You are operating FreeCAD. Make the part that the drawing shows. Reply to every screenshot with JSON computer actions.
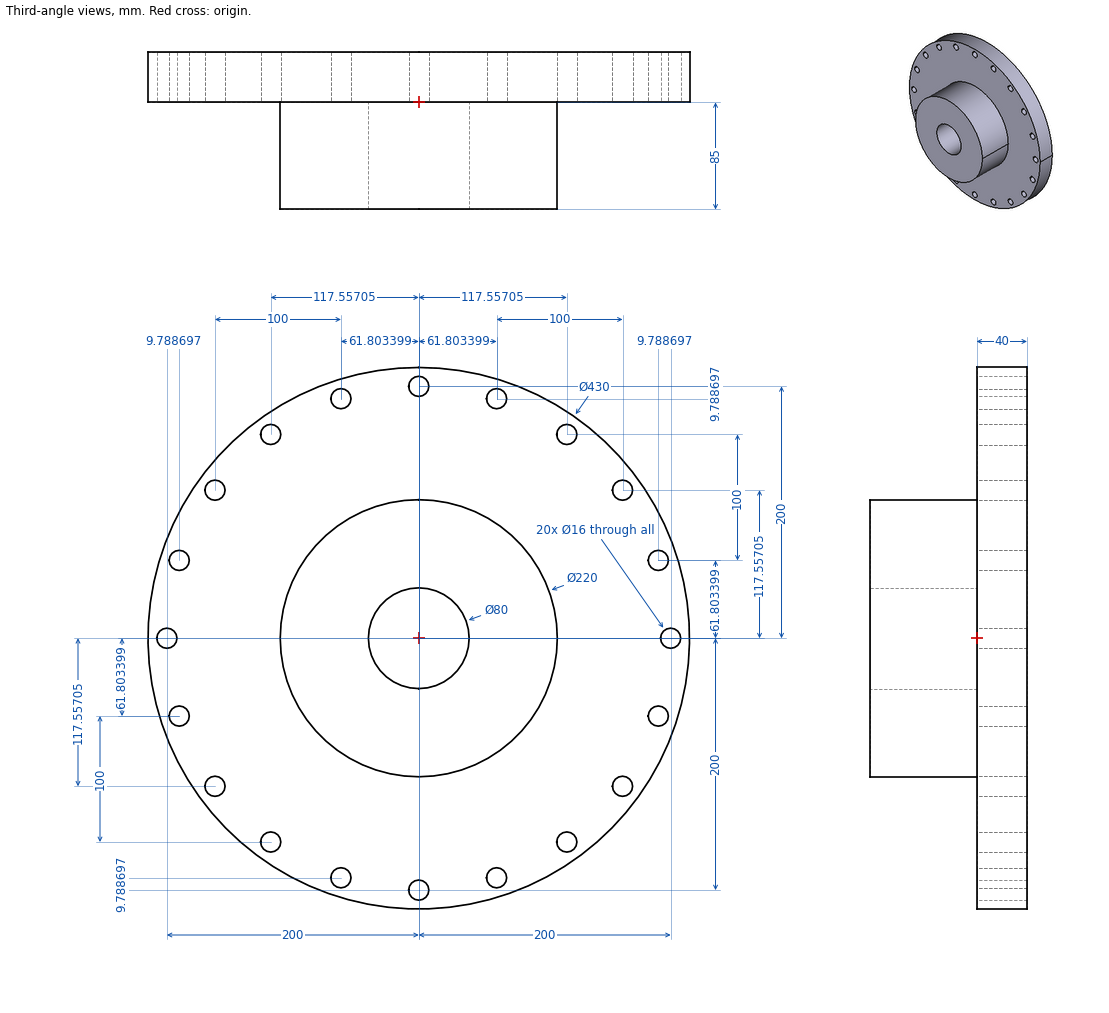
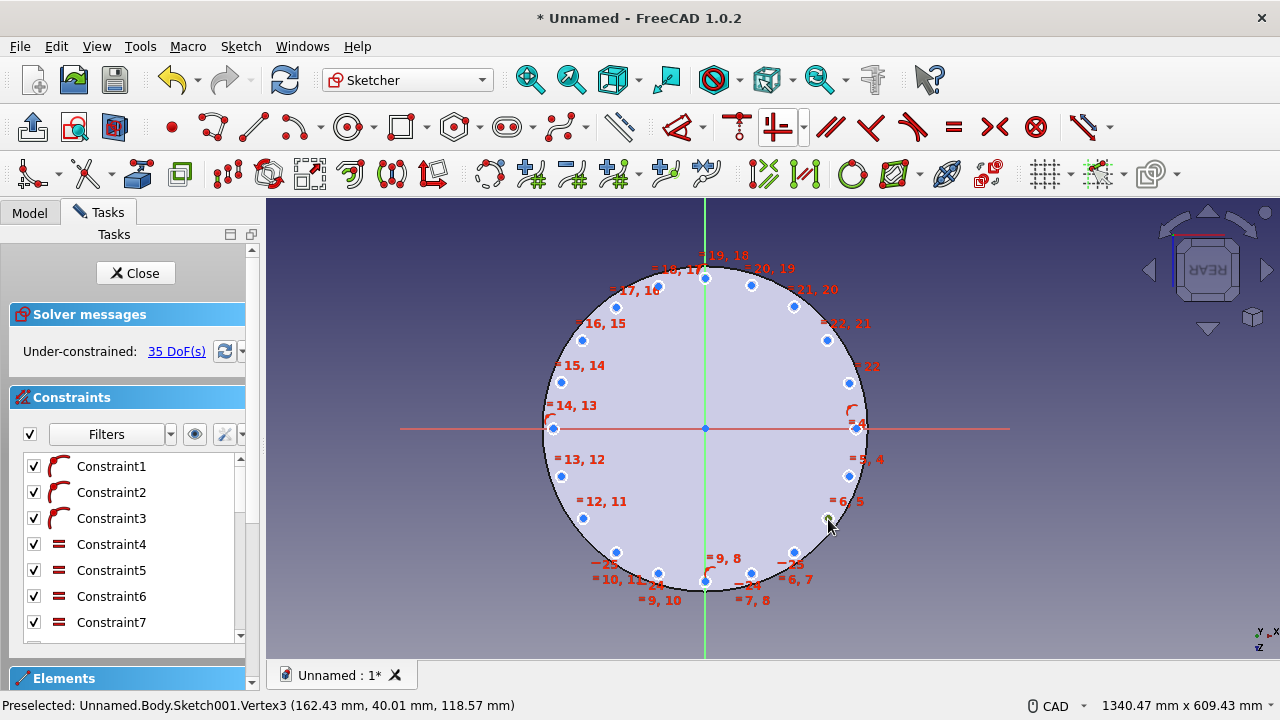
{"action": "left_click", "coordinate": [583, 519]}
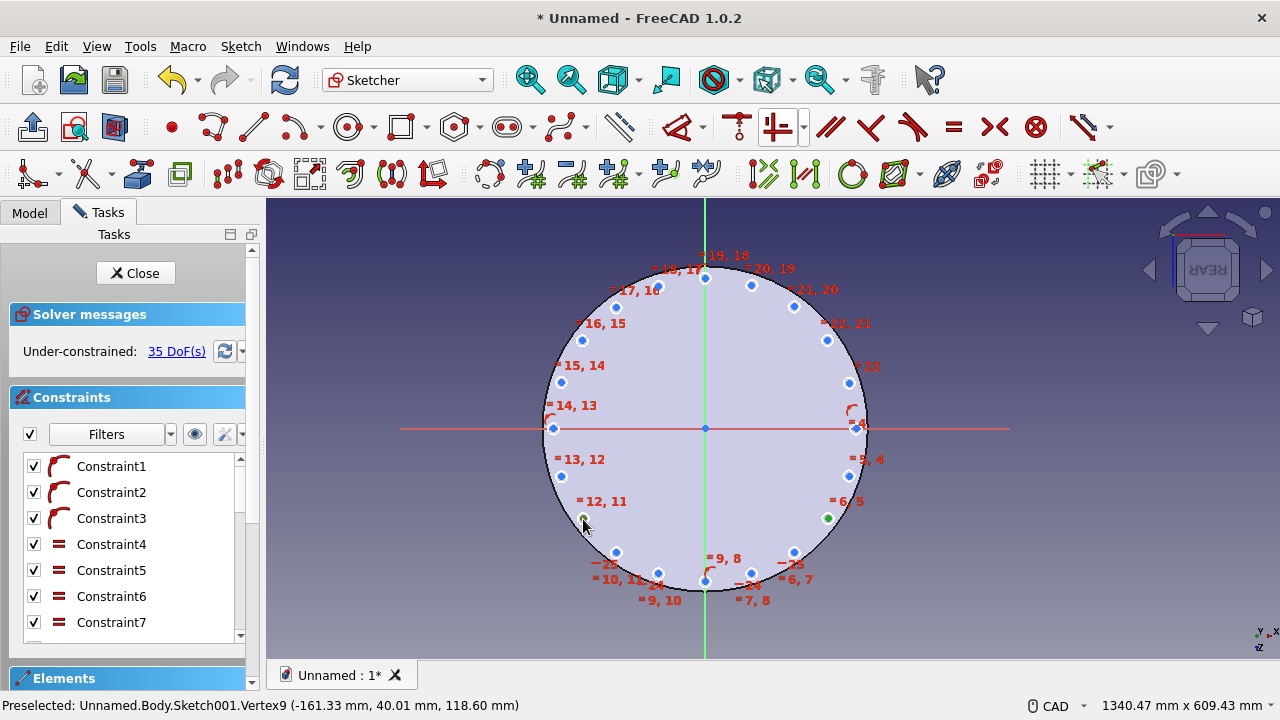
{"action": "left_click", "coordinate": [804, 128]}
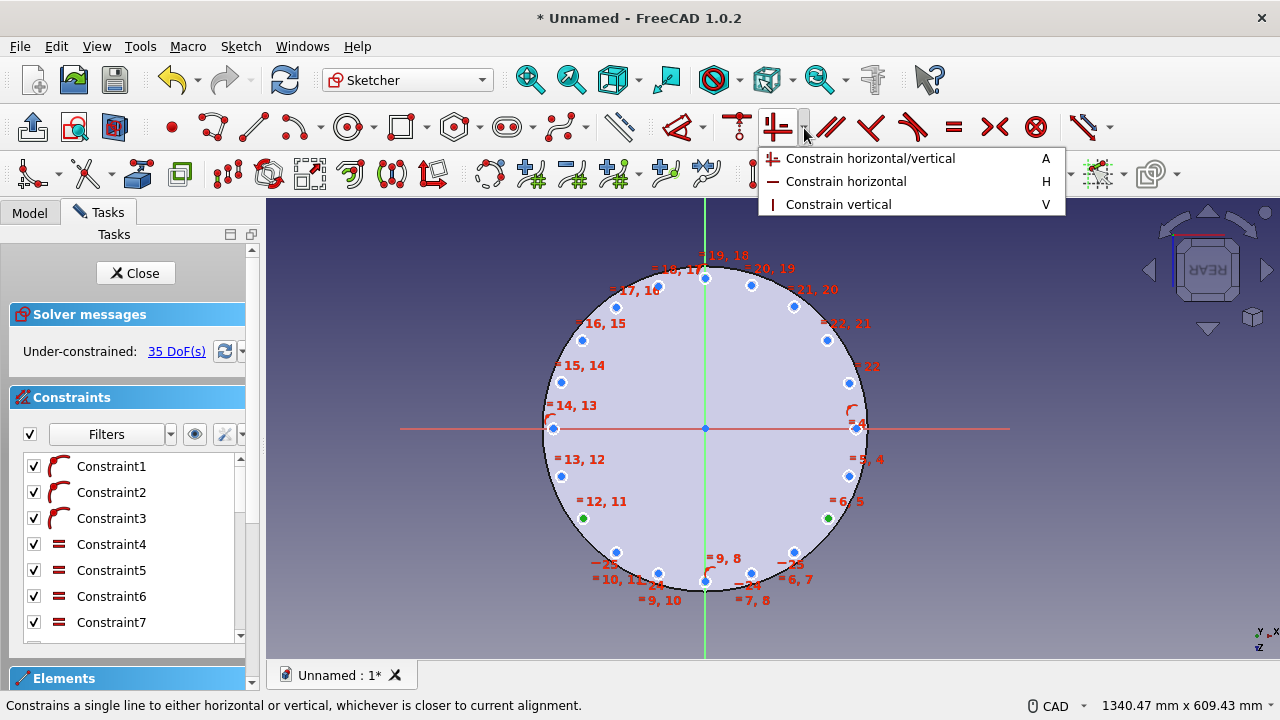
{"action": "left_click", "coordinate": [912, 182]}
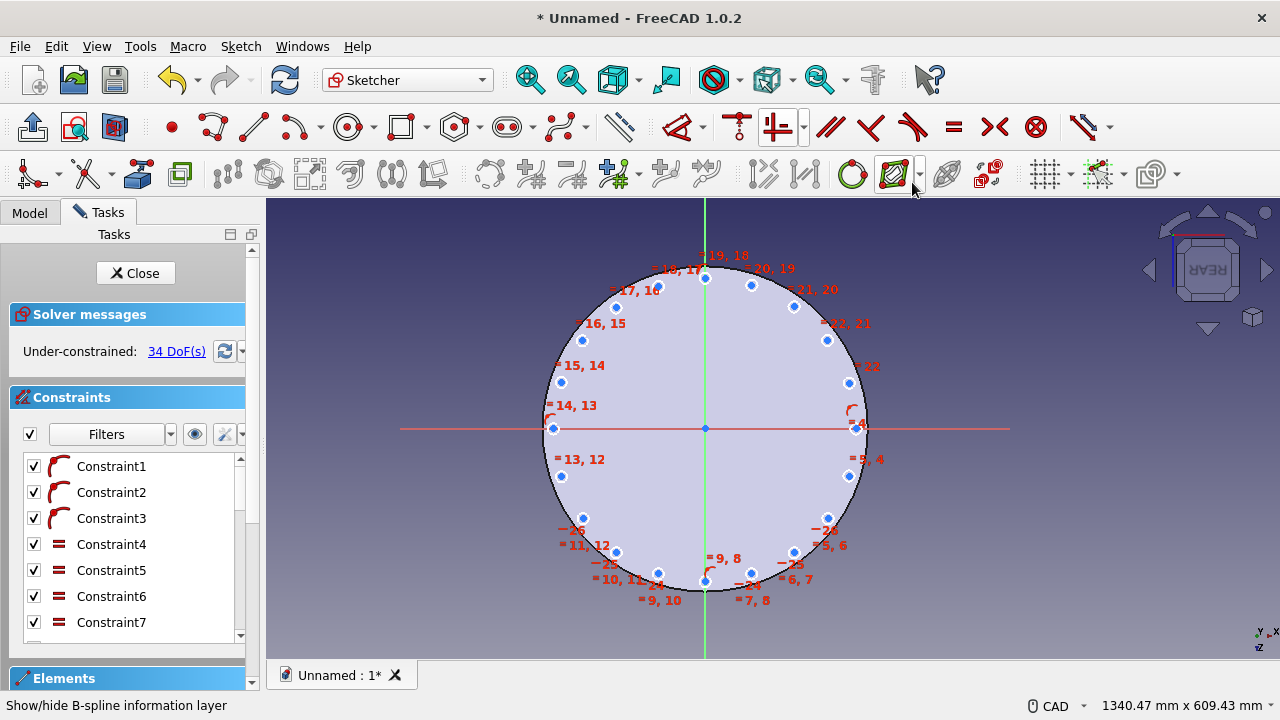
{"action": "left_click", "coordinate": [562, 477]}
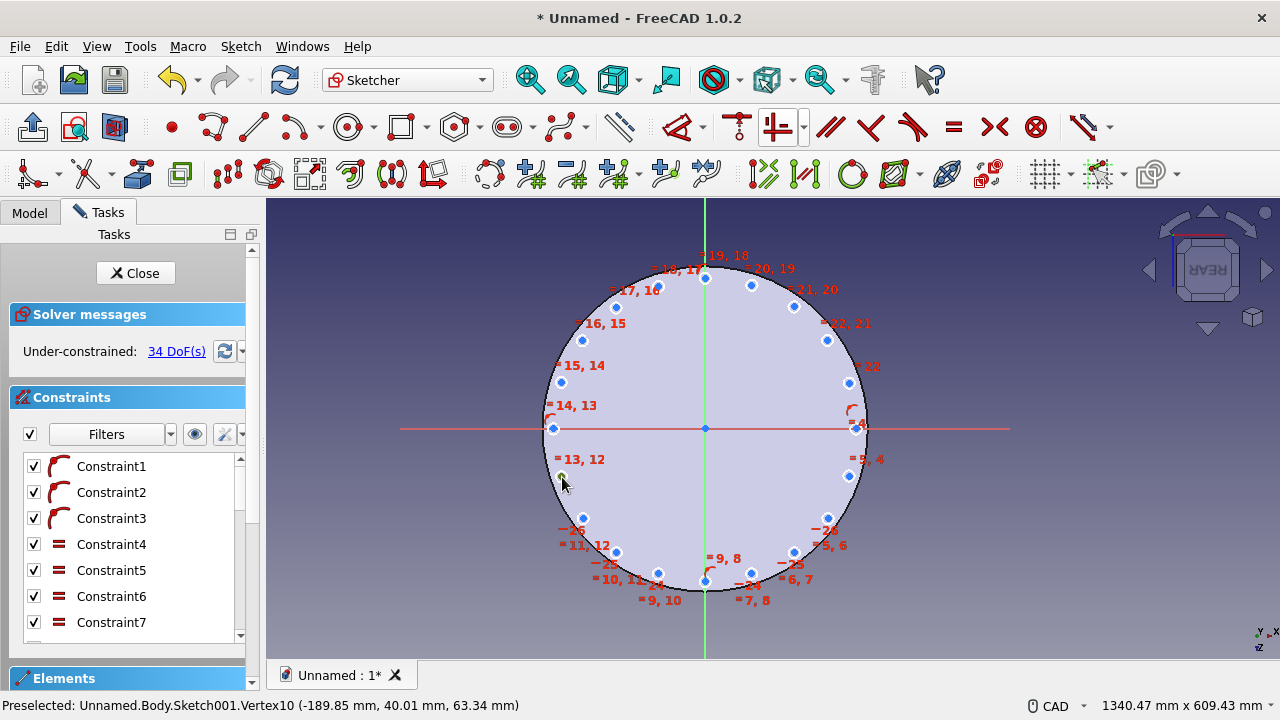
{"action": "left_click", "coordinate": [561, 383]}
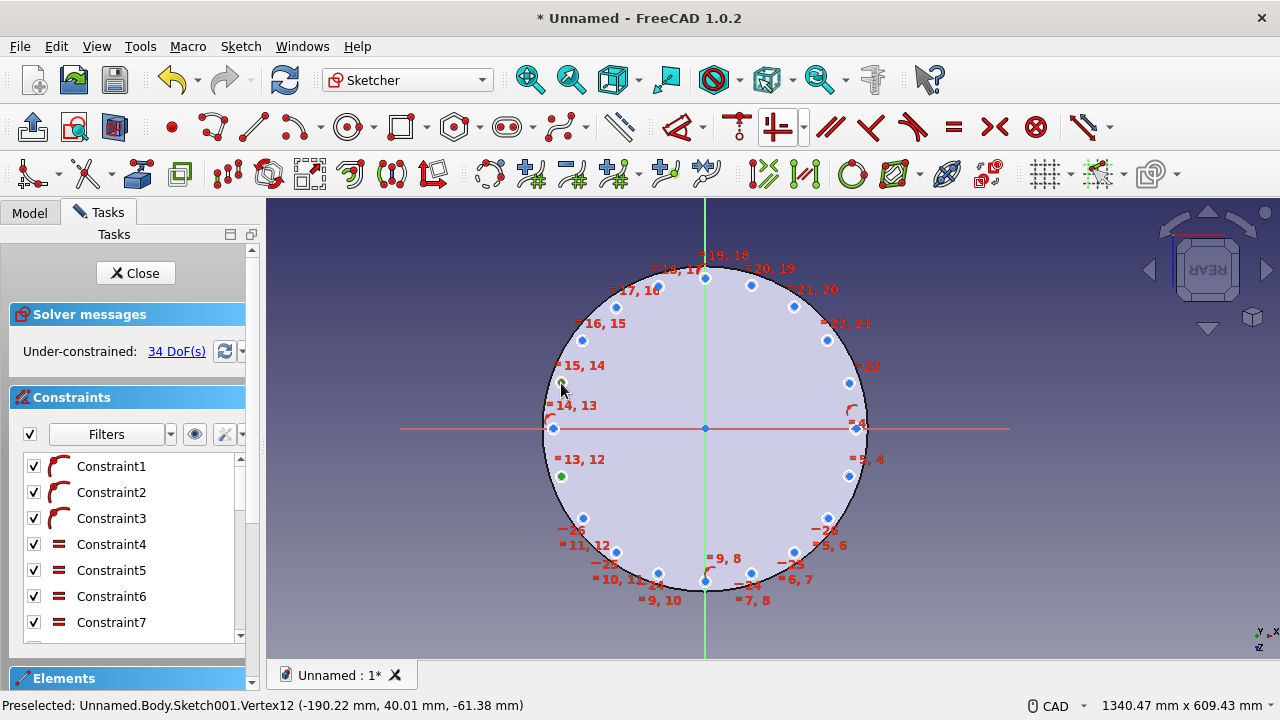
{"action": "key", "text": "v"}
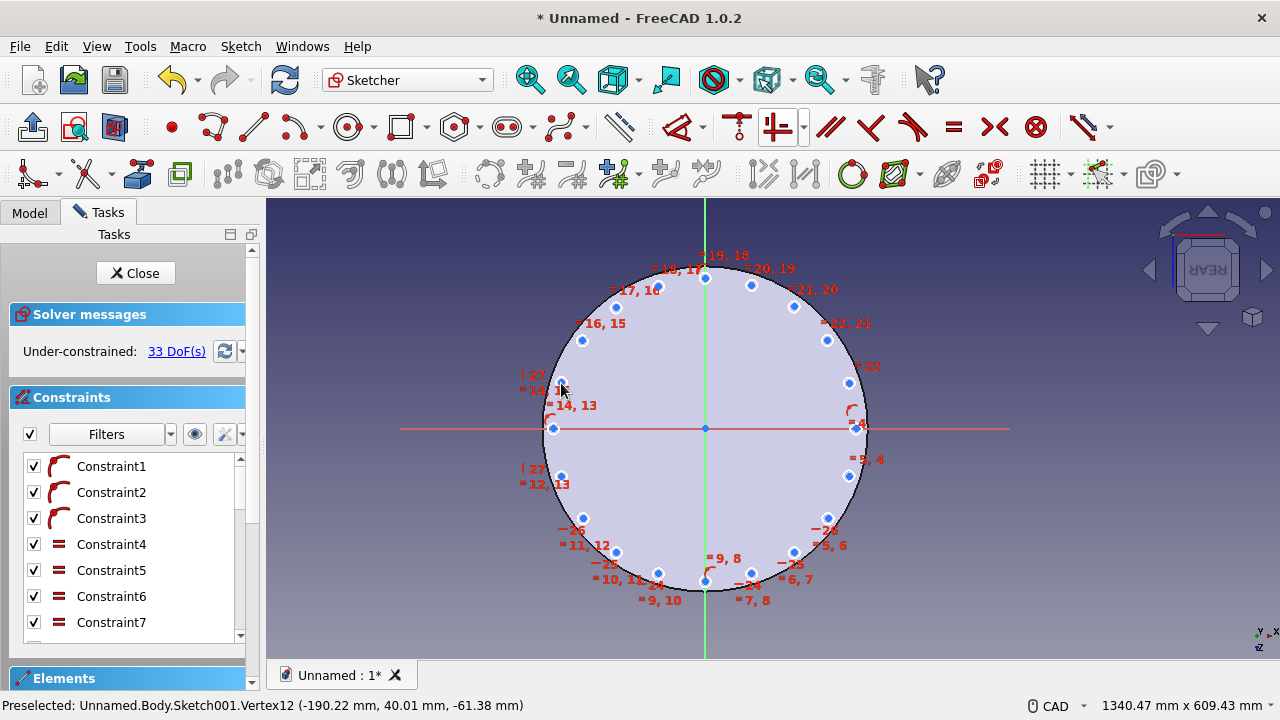
{"action": "left_click", "coordinate": [583, 519]}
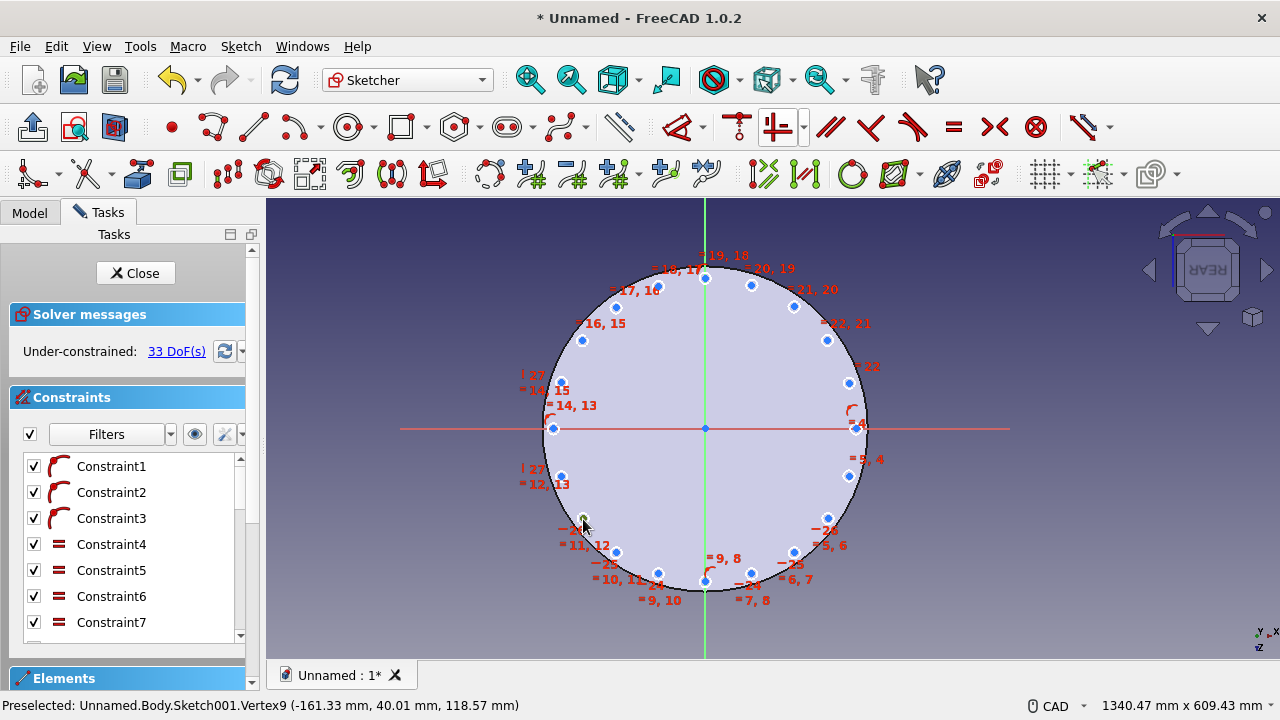
{"action": "left_click", "coordinate": [582, 341]}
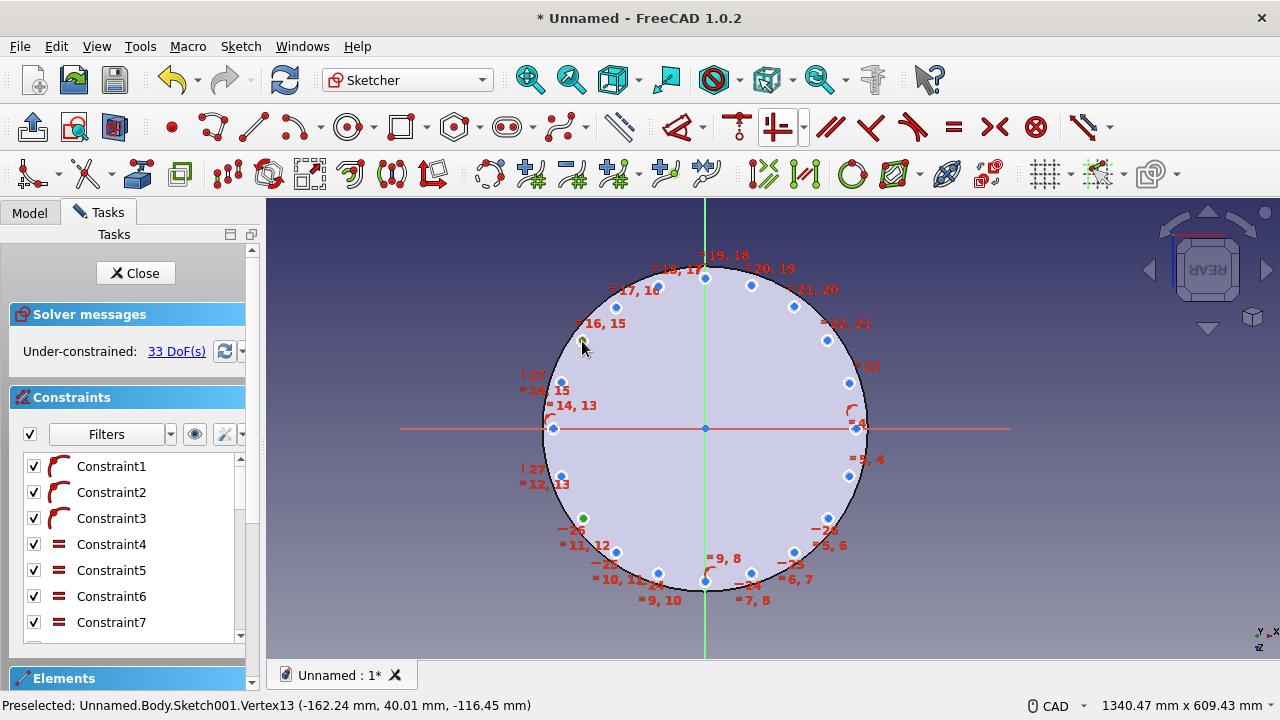
{"action": "key", "text": "v"}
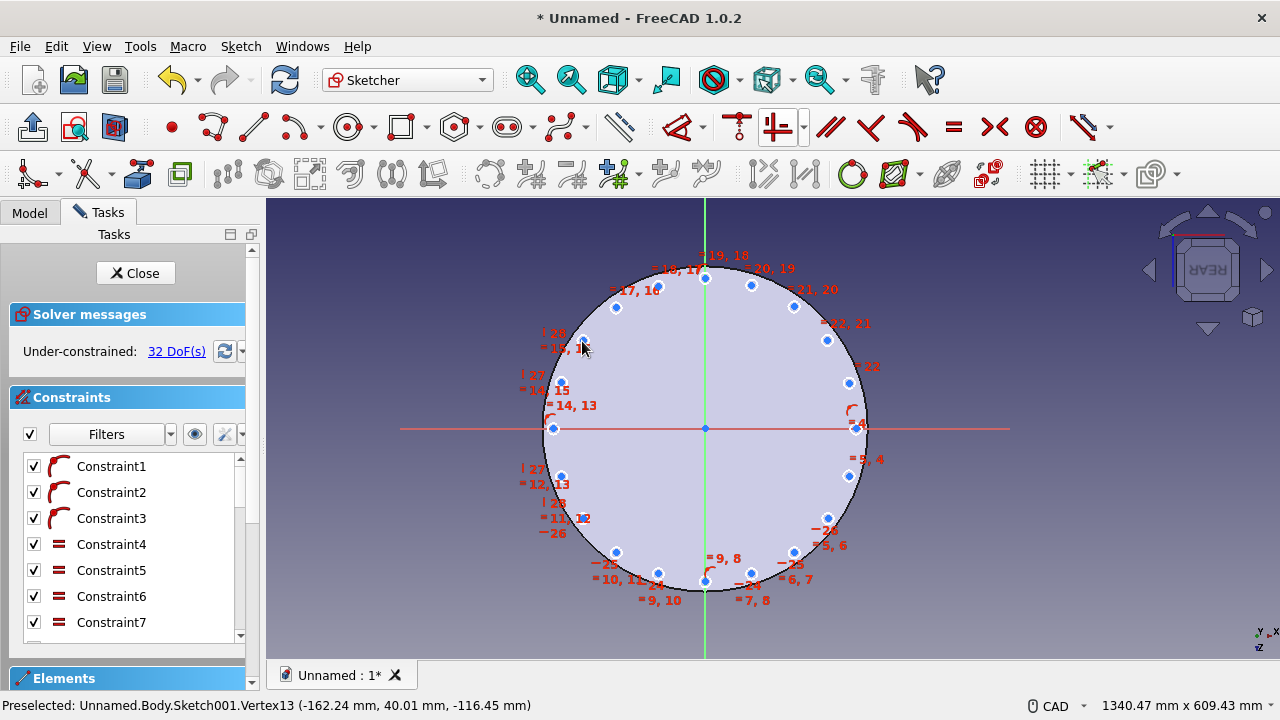
{"action": "left_click", "coordinate": [616, 553]}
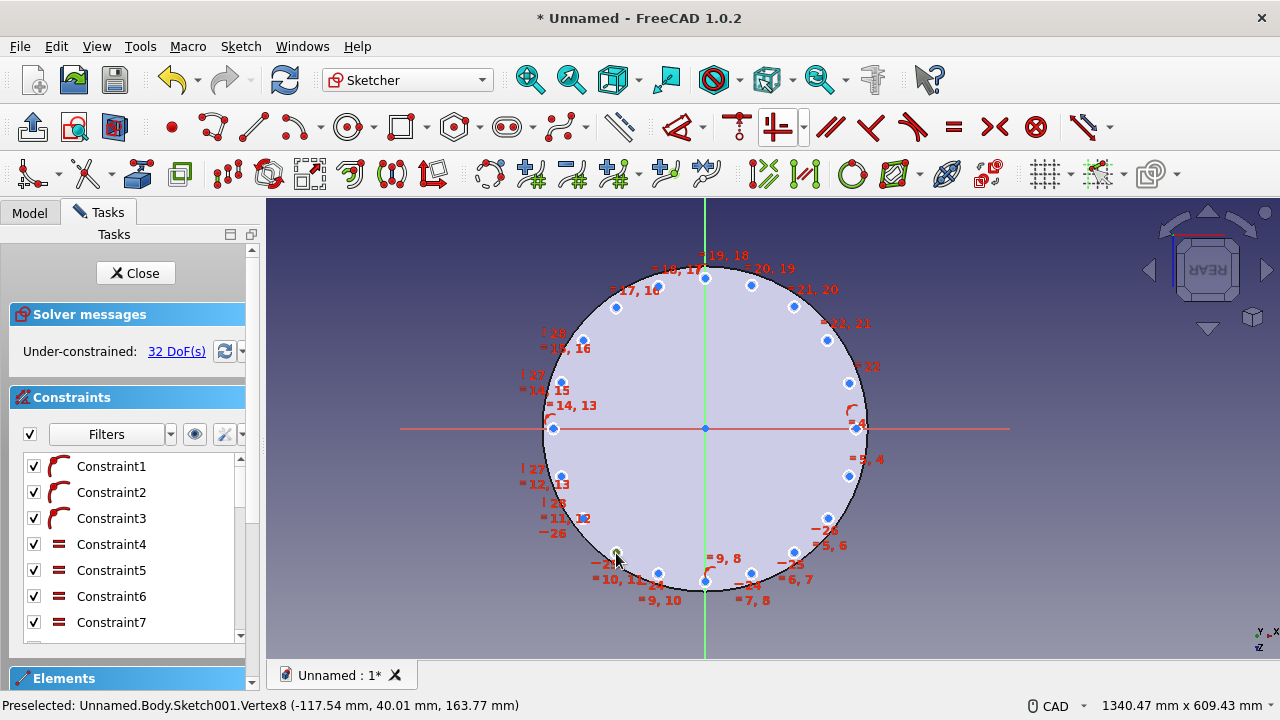
{"action": "left_click", "coordinate": [616, 308]}